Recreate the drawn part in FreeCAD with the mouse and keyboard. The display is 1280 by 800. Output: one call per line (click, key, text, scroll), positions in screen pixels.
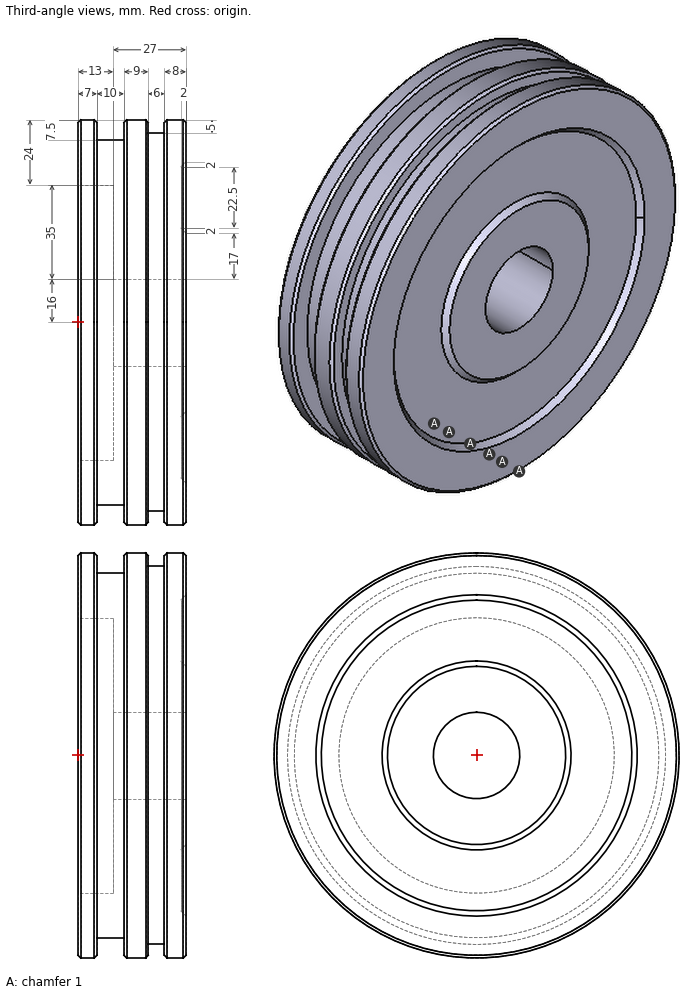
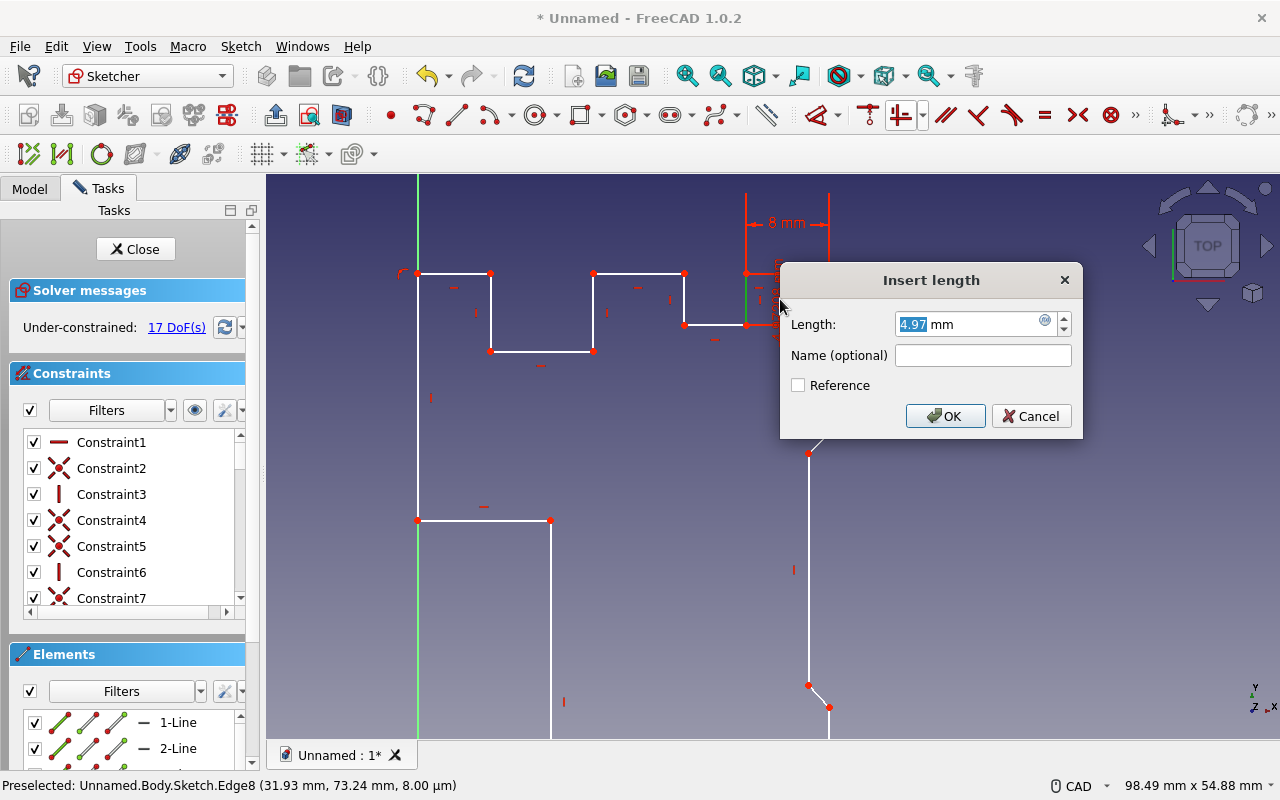
text(5)
key(Return)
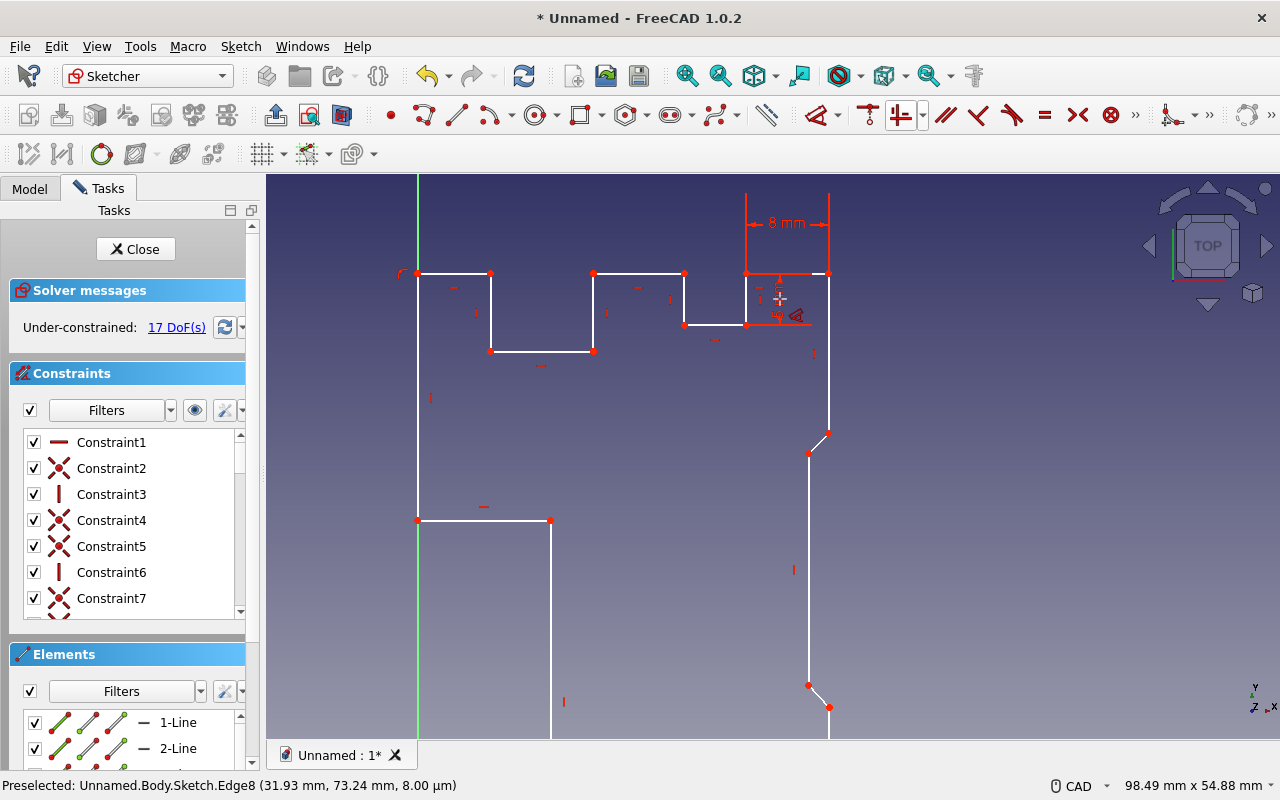
click(728, 325)
click(701, 291)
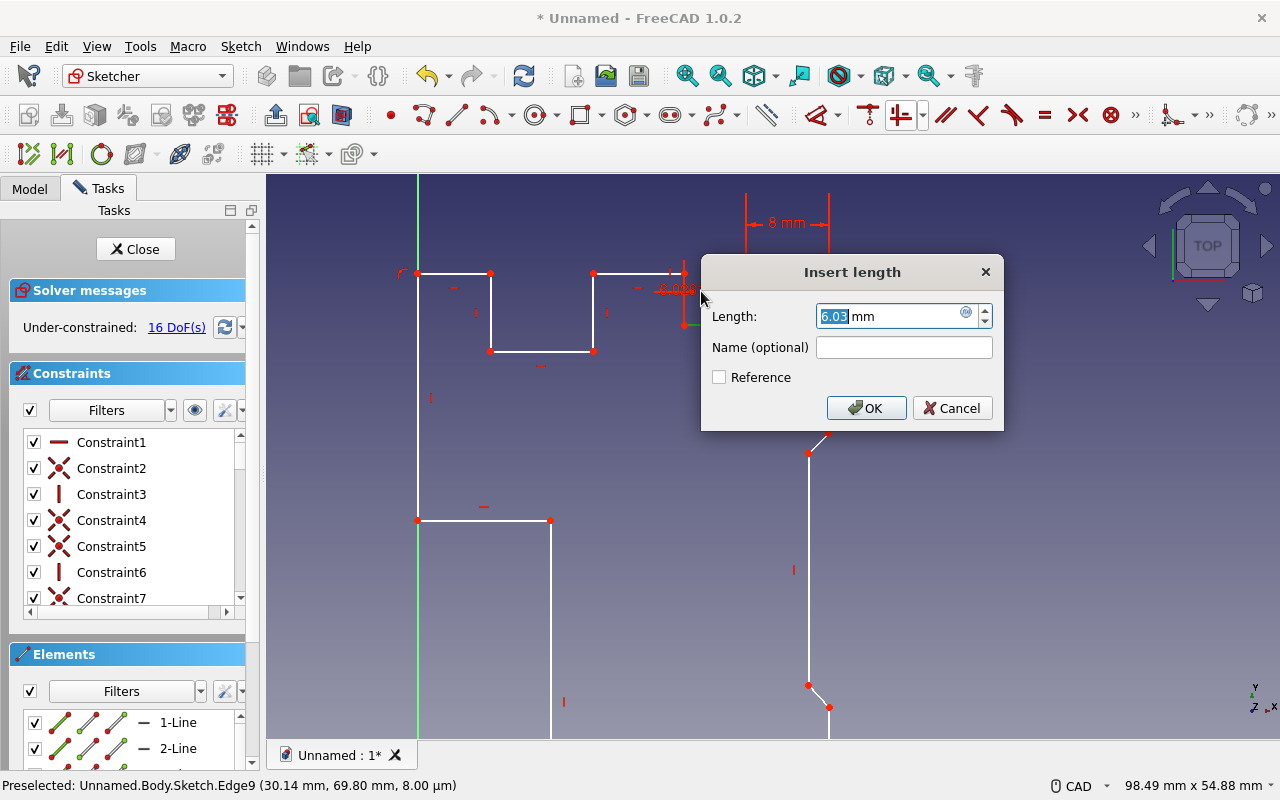
text(6)
key(Return)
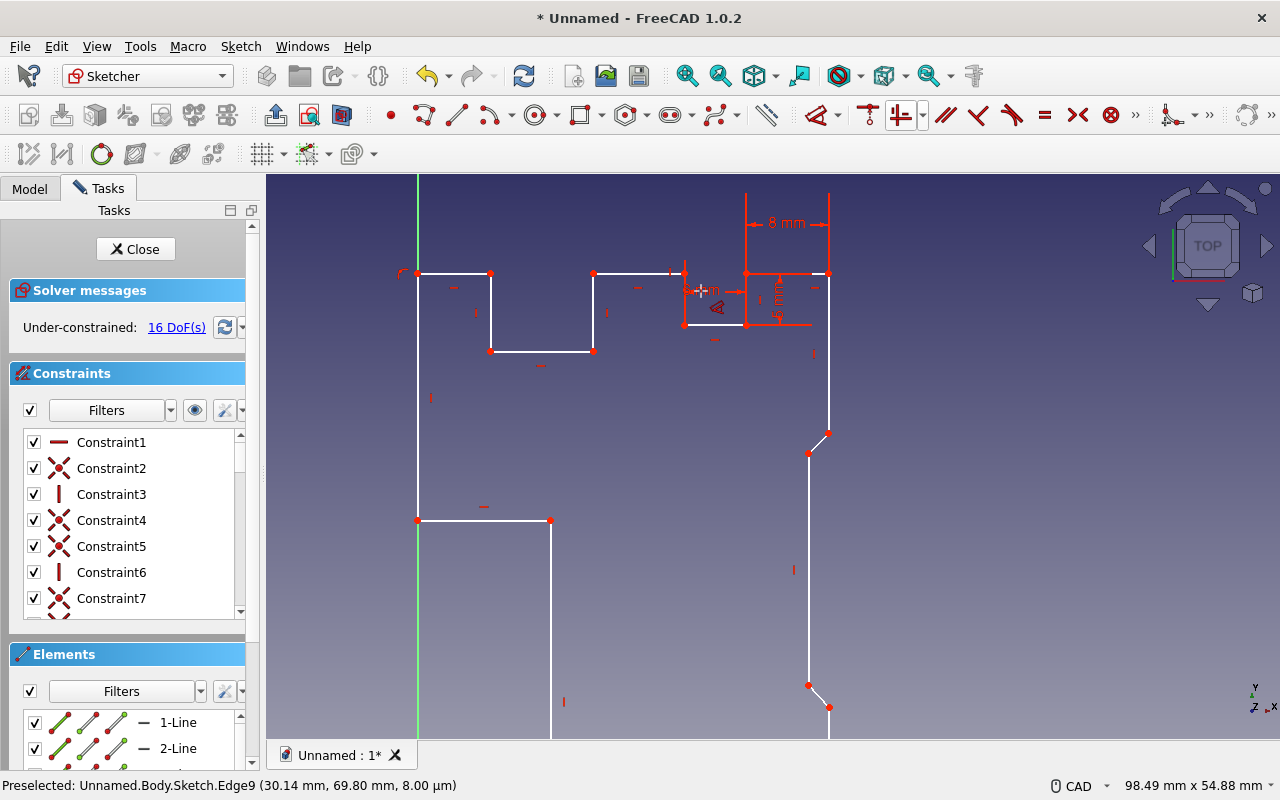
click(685, 310)
click(651, 311)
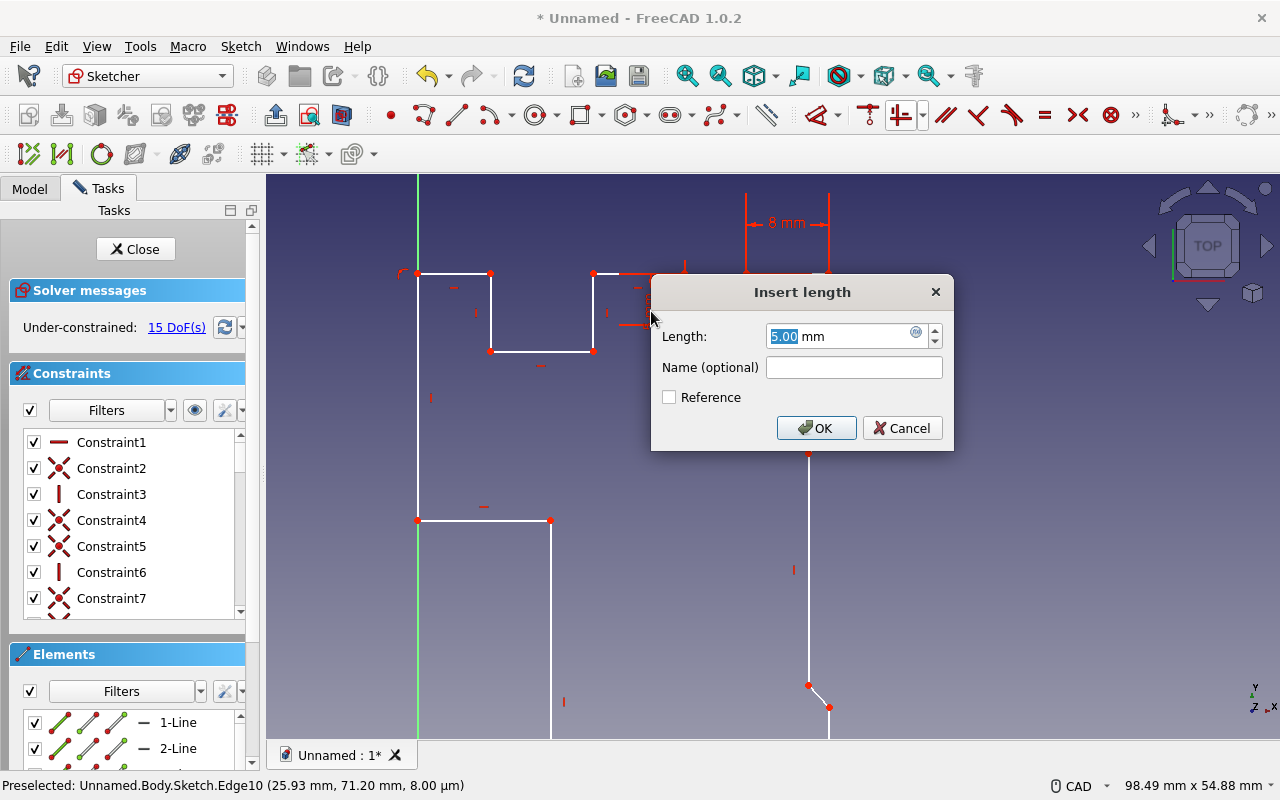
text(5)
key(Return)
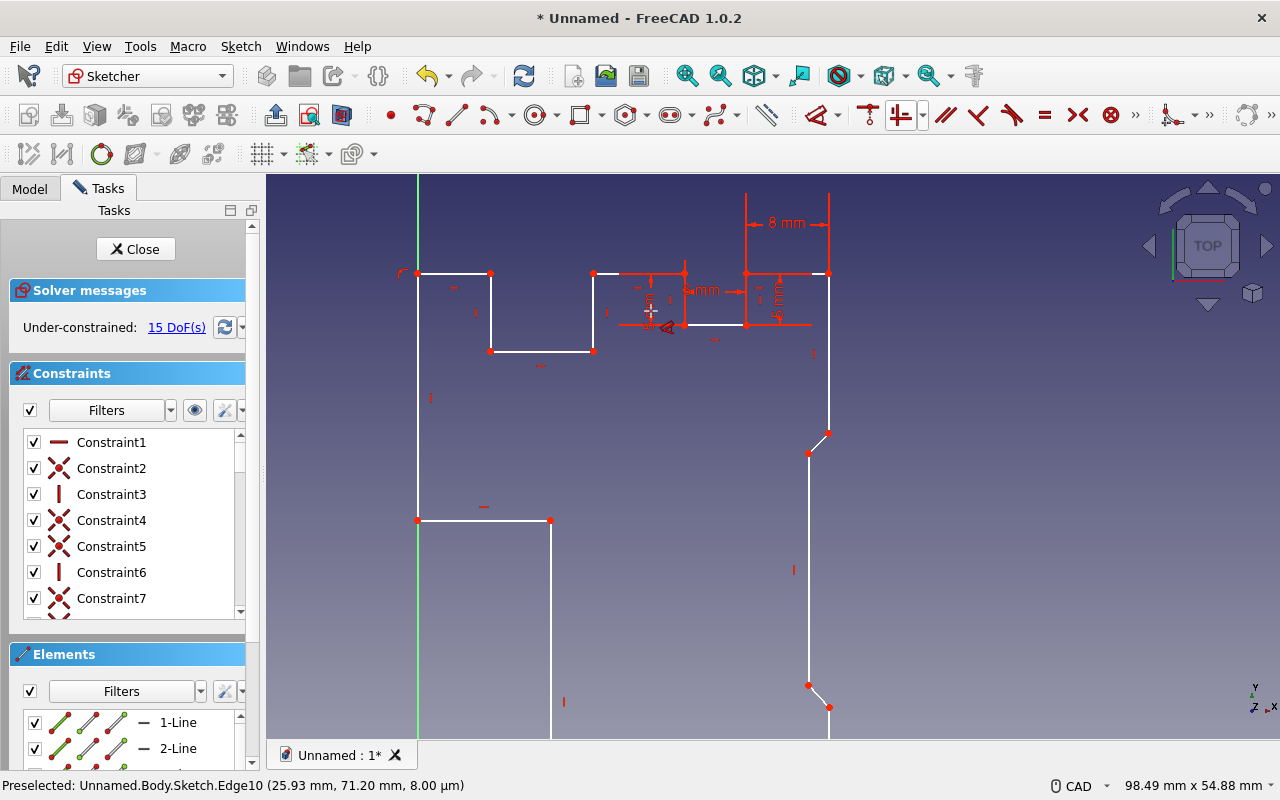
click(657, 274)
click(639, 240)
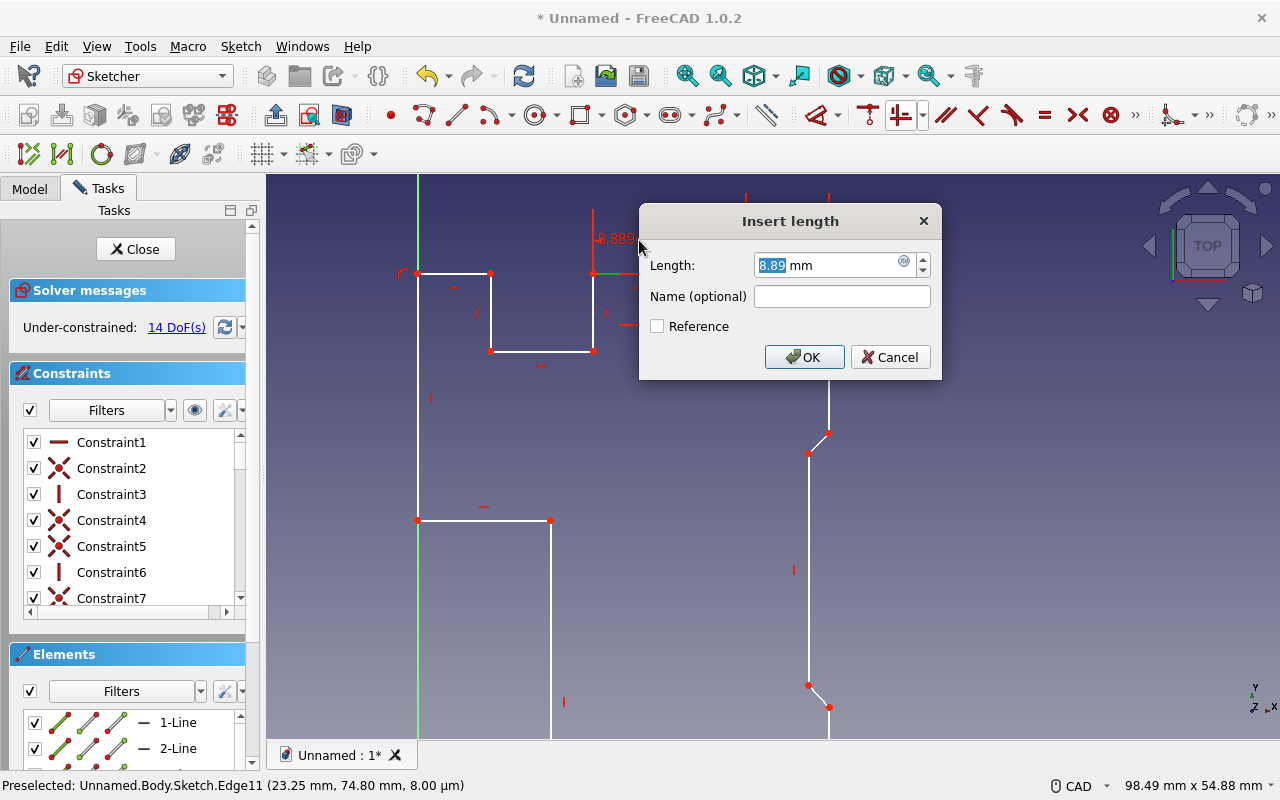
text(9)
key(Return)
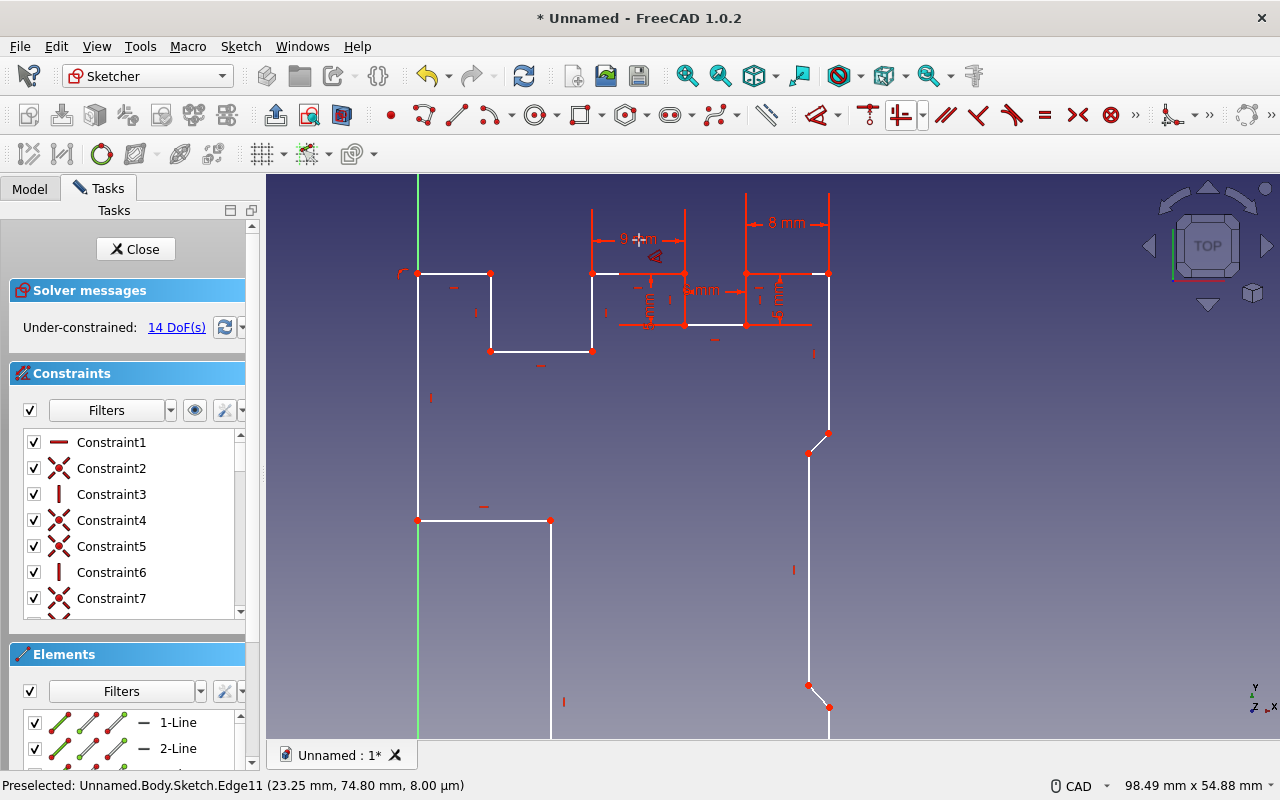
click(469, 274)
click(454, 240)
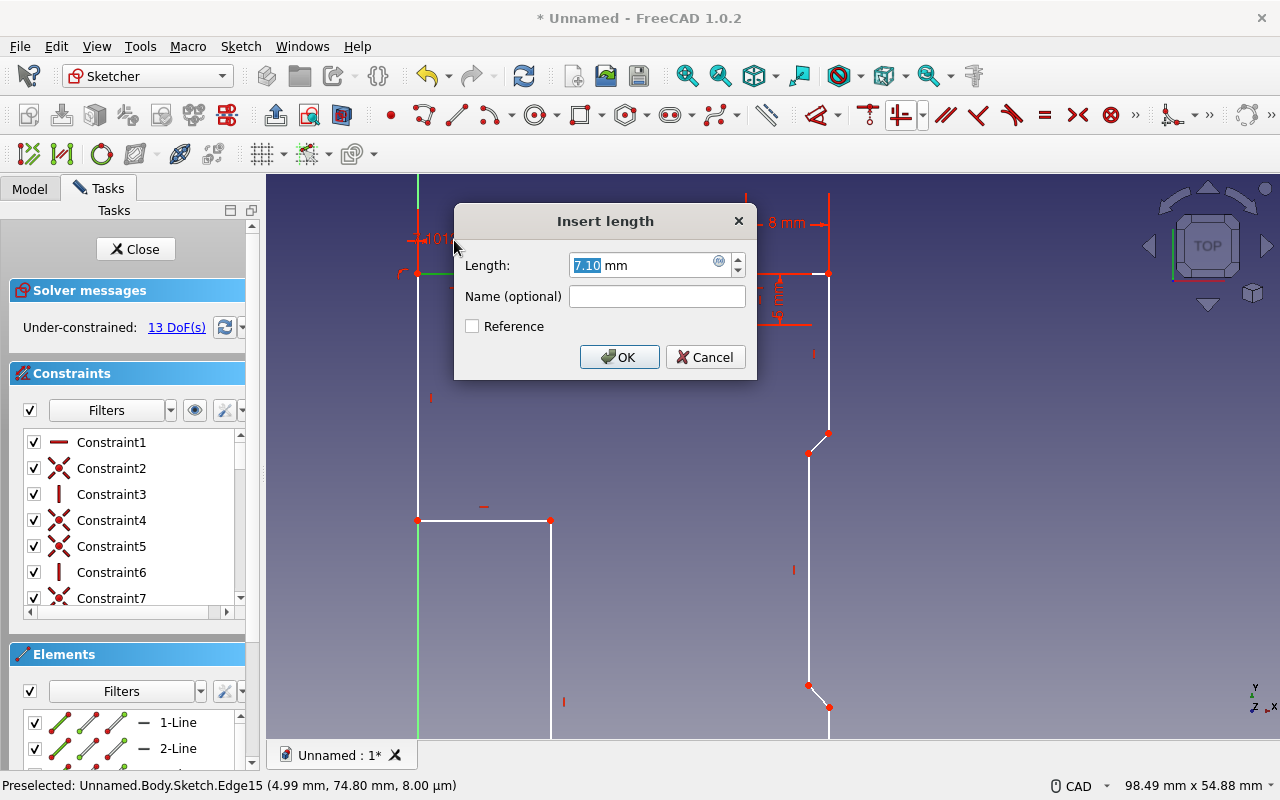
text(7)
key(Return)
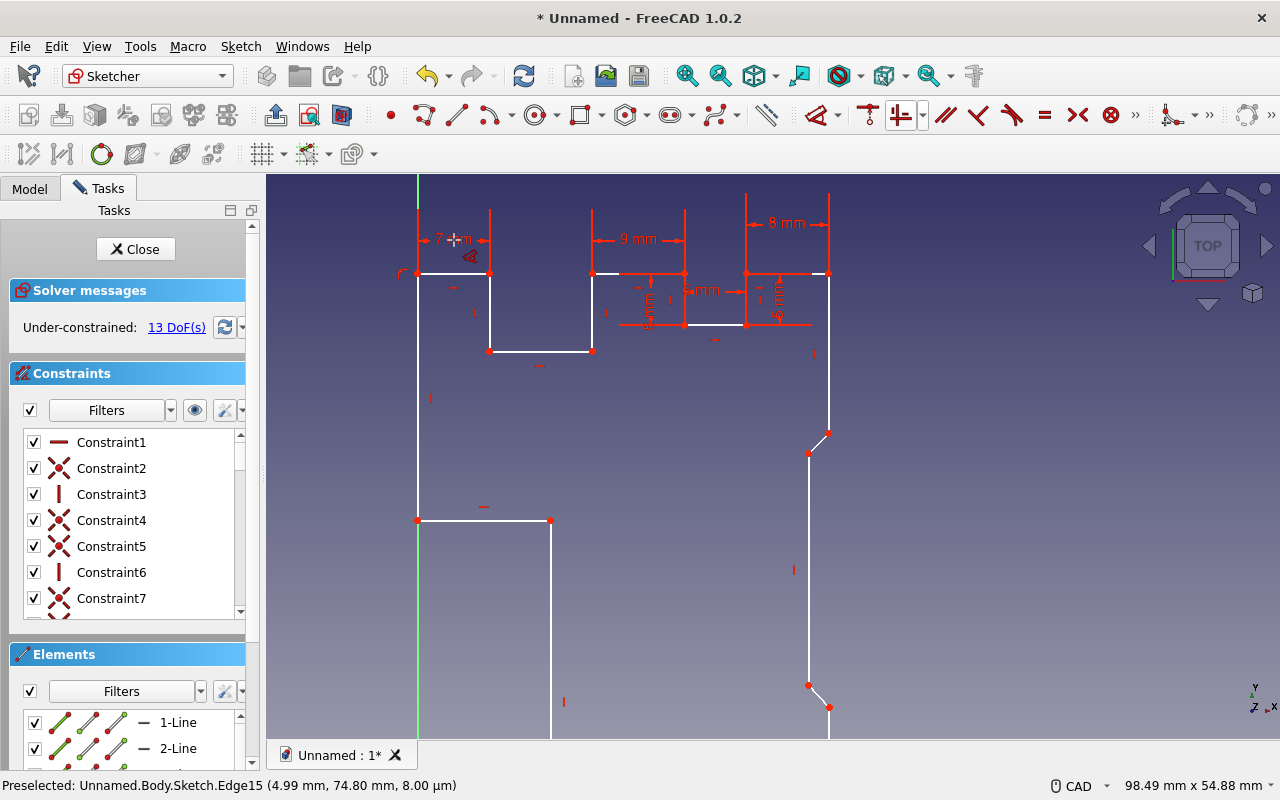
scroll(771, 292, down, 4)